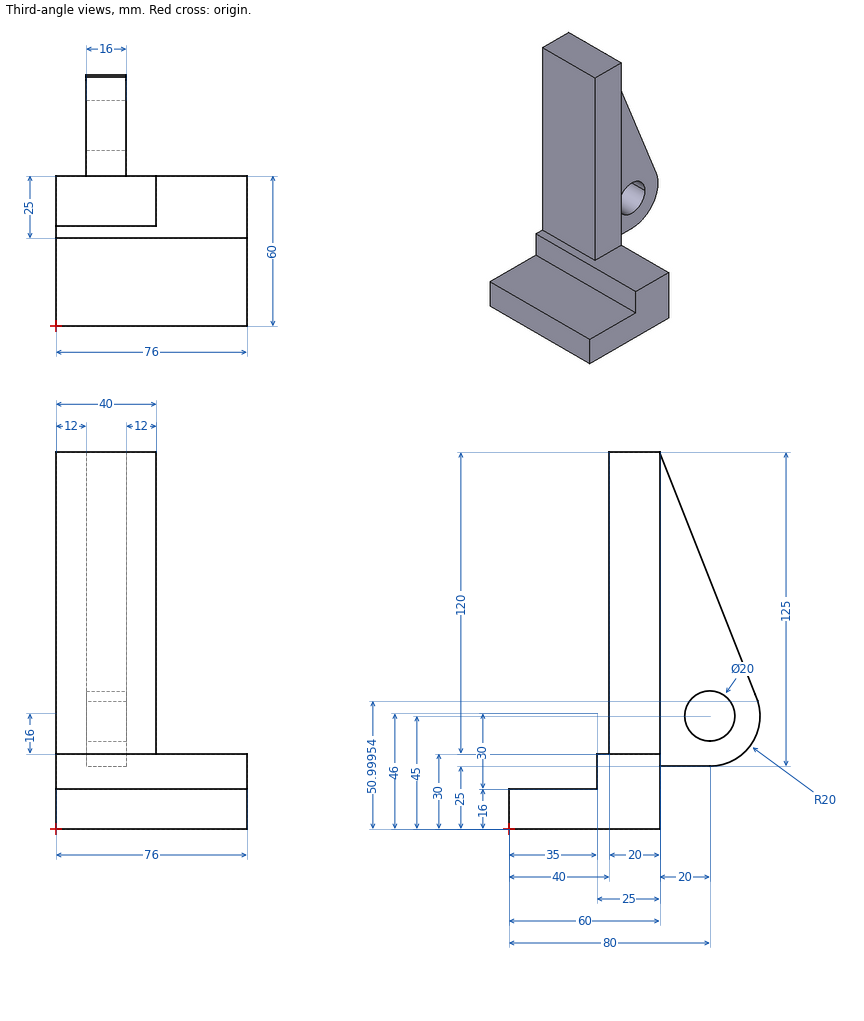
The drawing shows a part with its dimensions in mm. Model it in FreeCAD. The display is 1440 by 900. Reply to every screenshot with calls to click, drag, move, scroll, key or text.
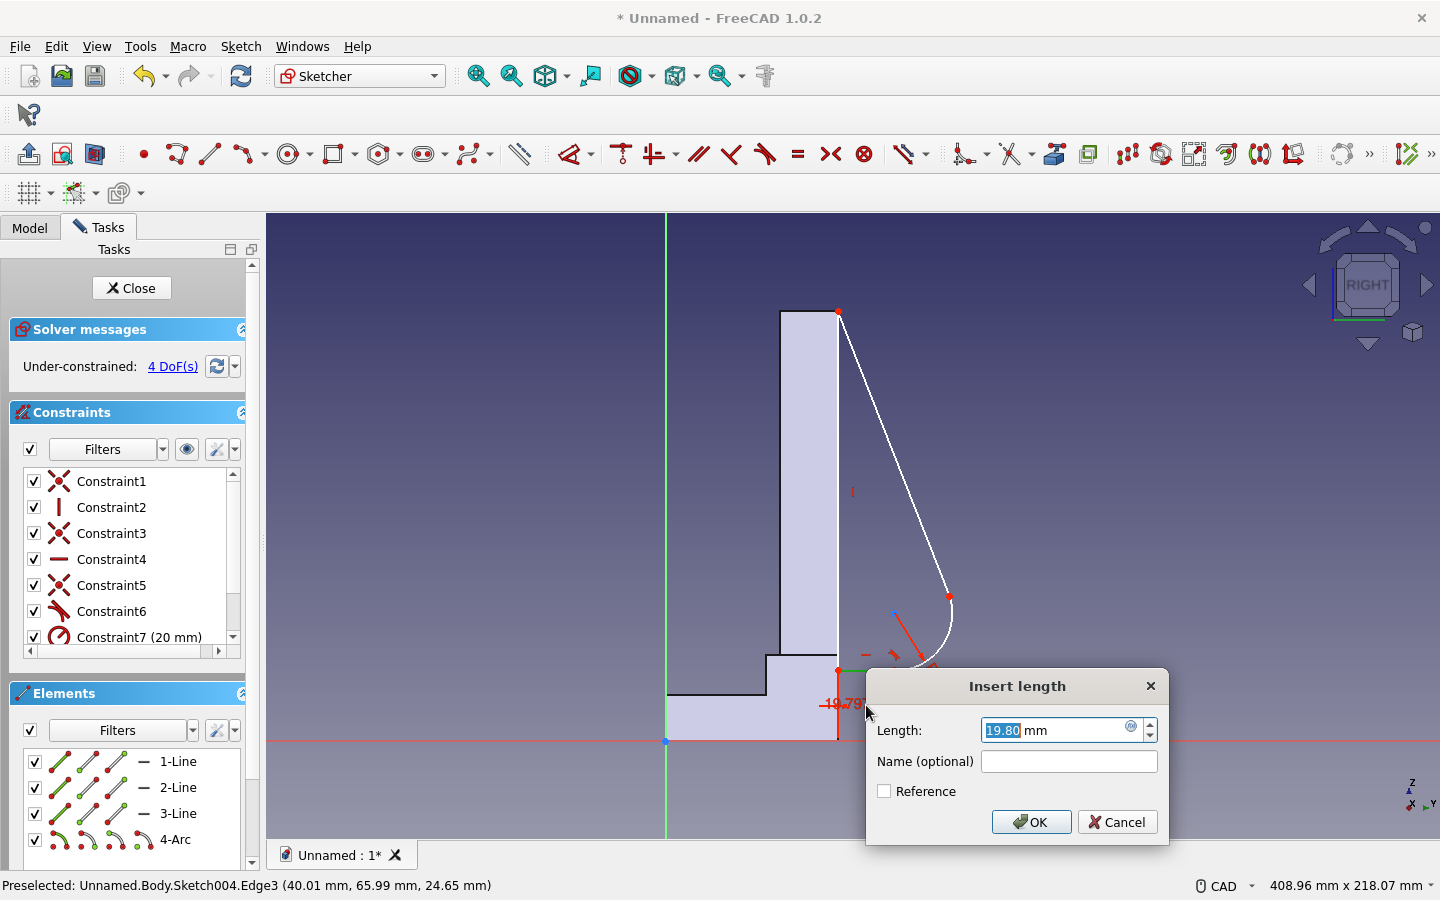
text(20)
key(Return)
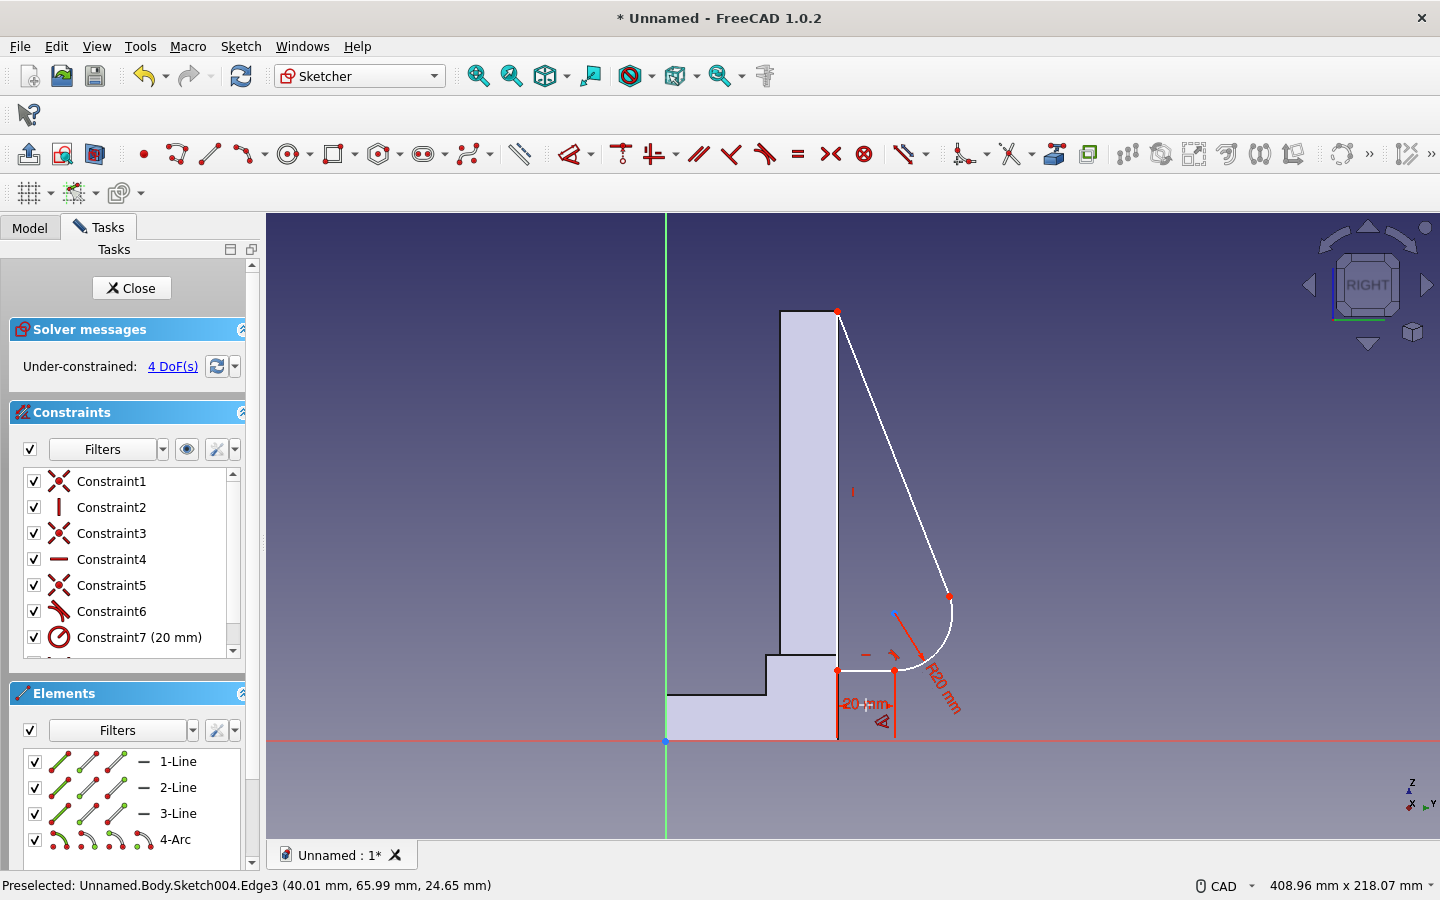
click(837, 420)
click(871, 491)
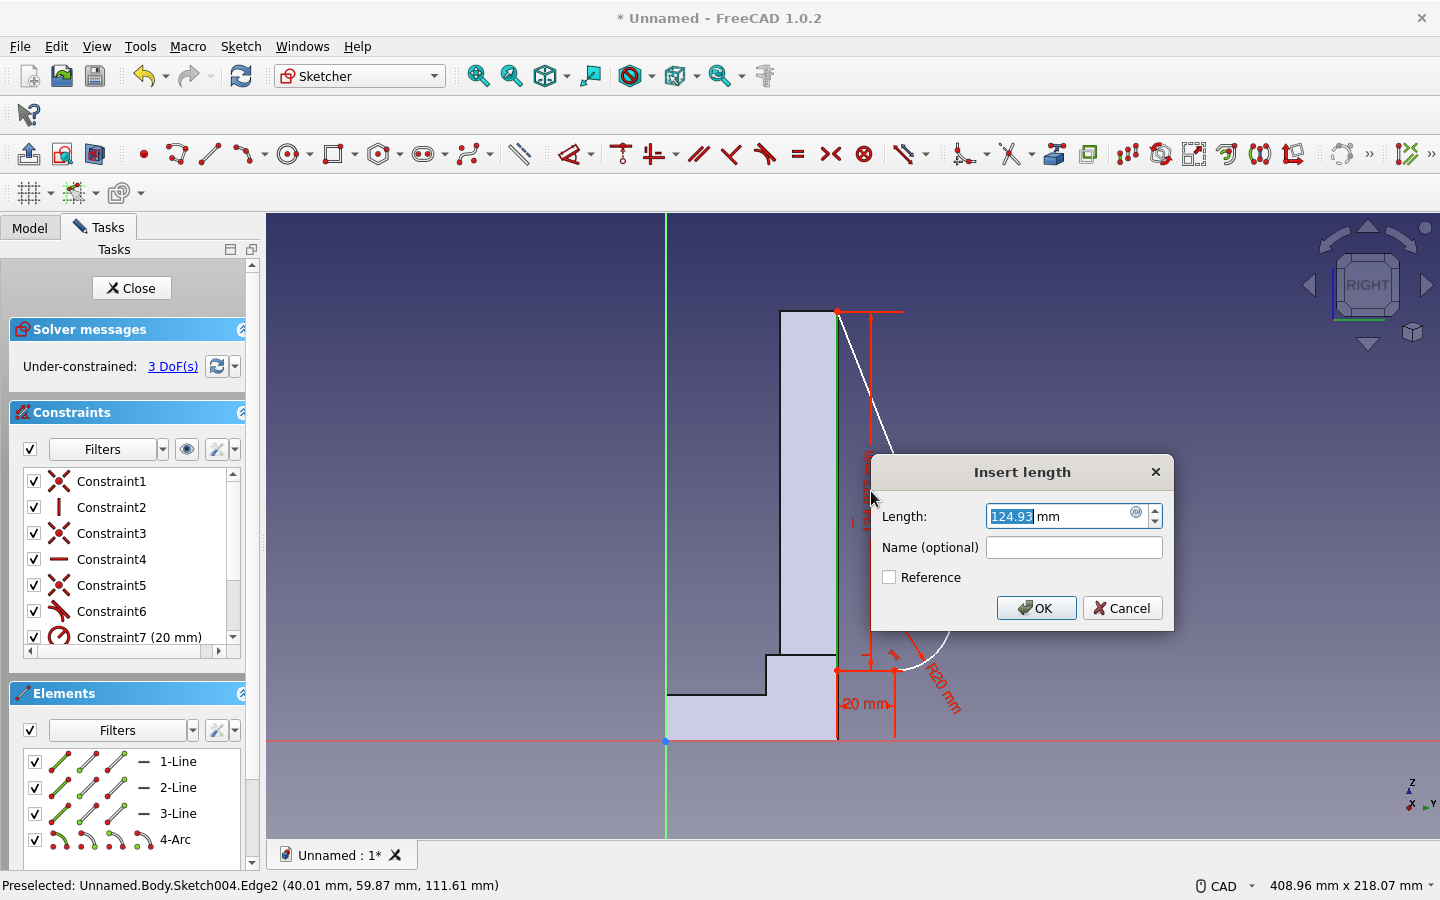
text(125)
key(Return)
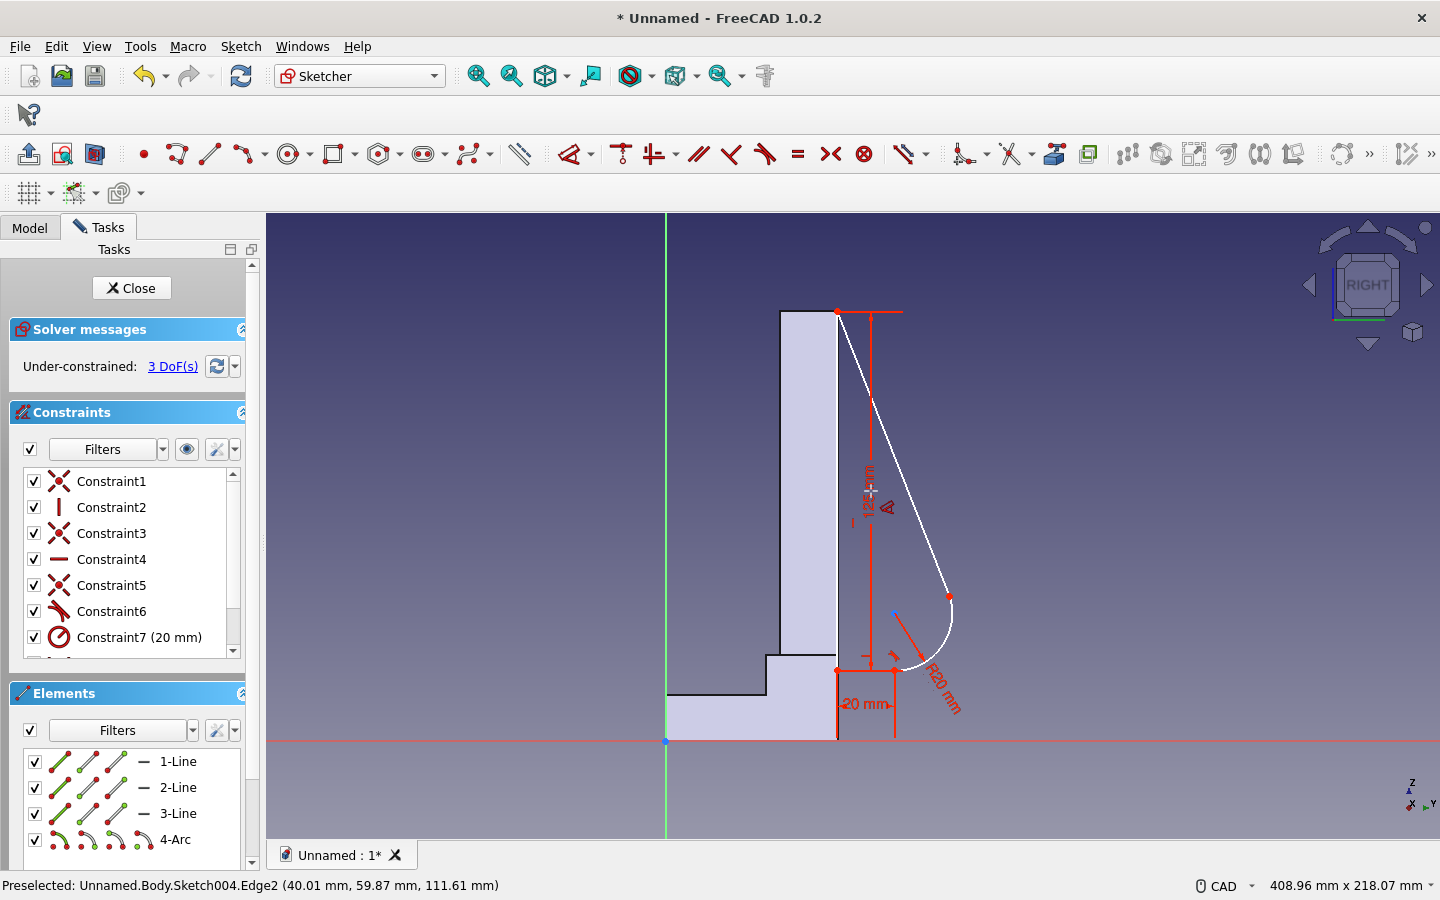
click(837, 312)
click(751, 775)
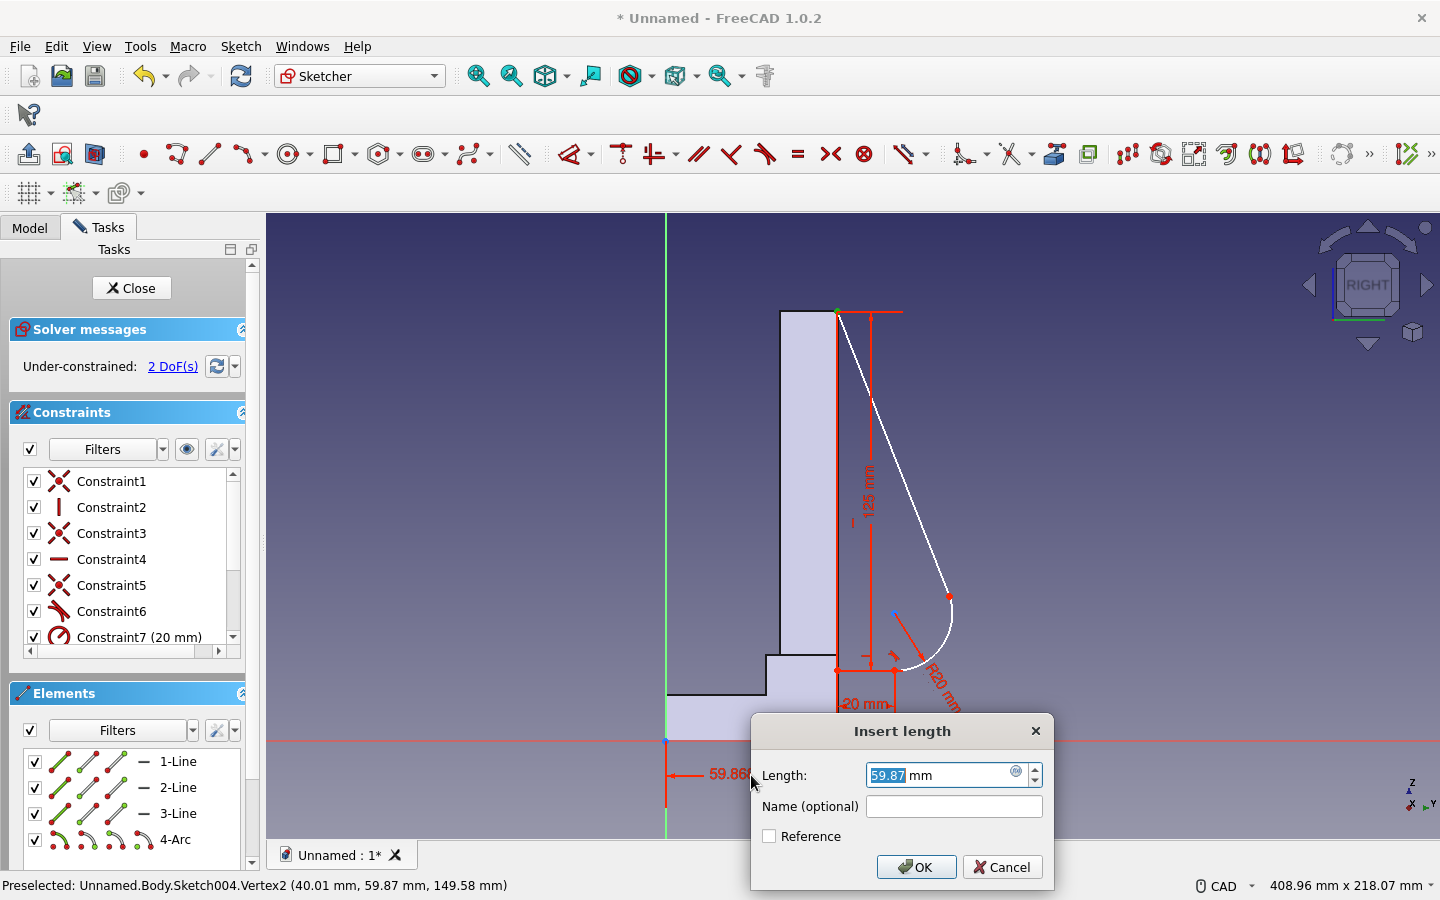
text(60)
key(Return)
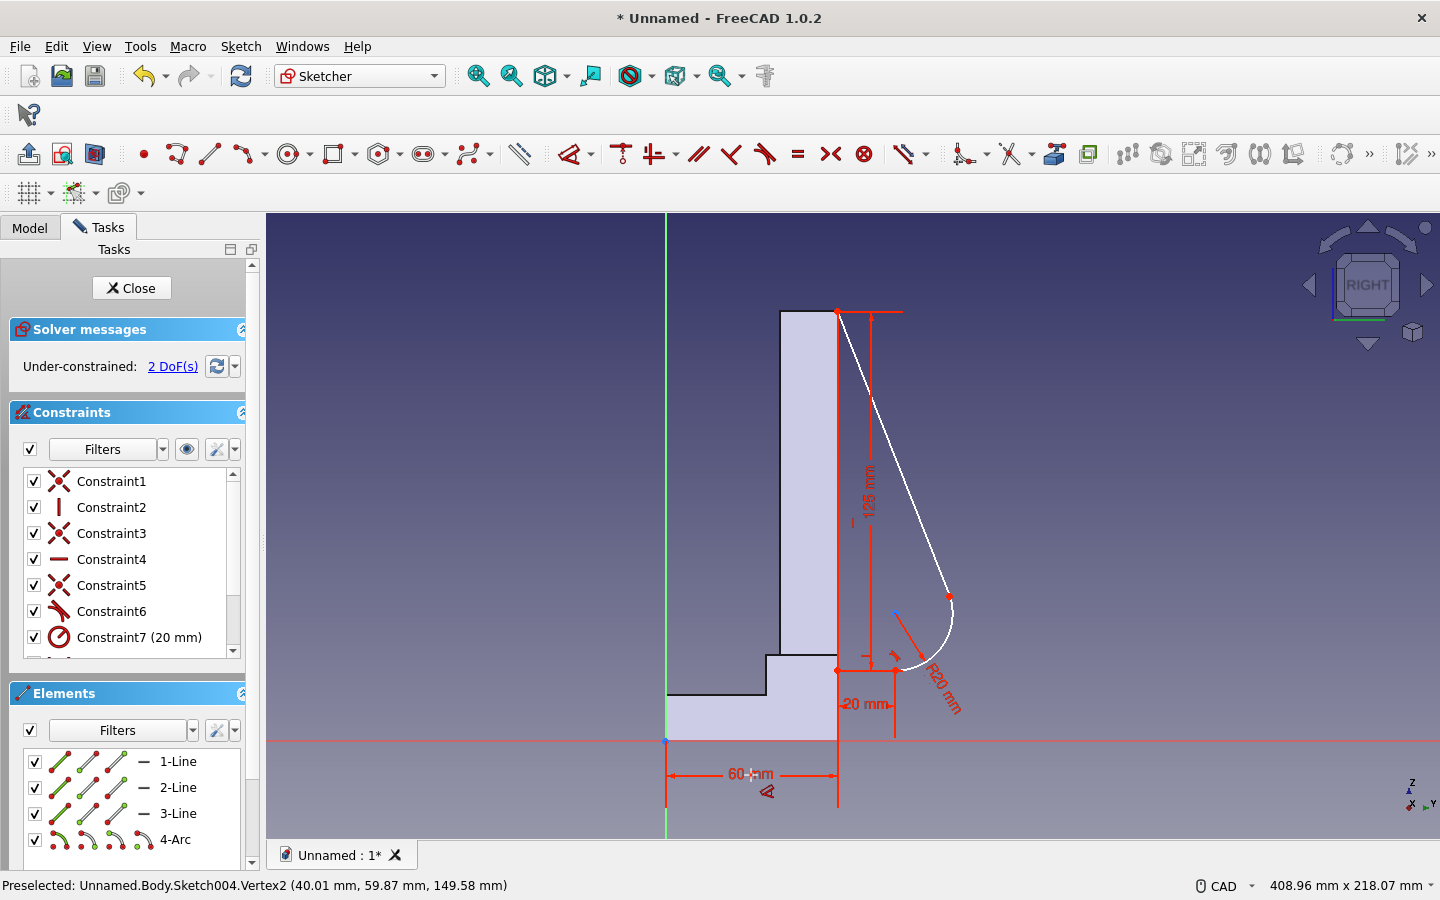
click(838, 671)
click(632, 706)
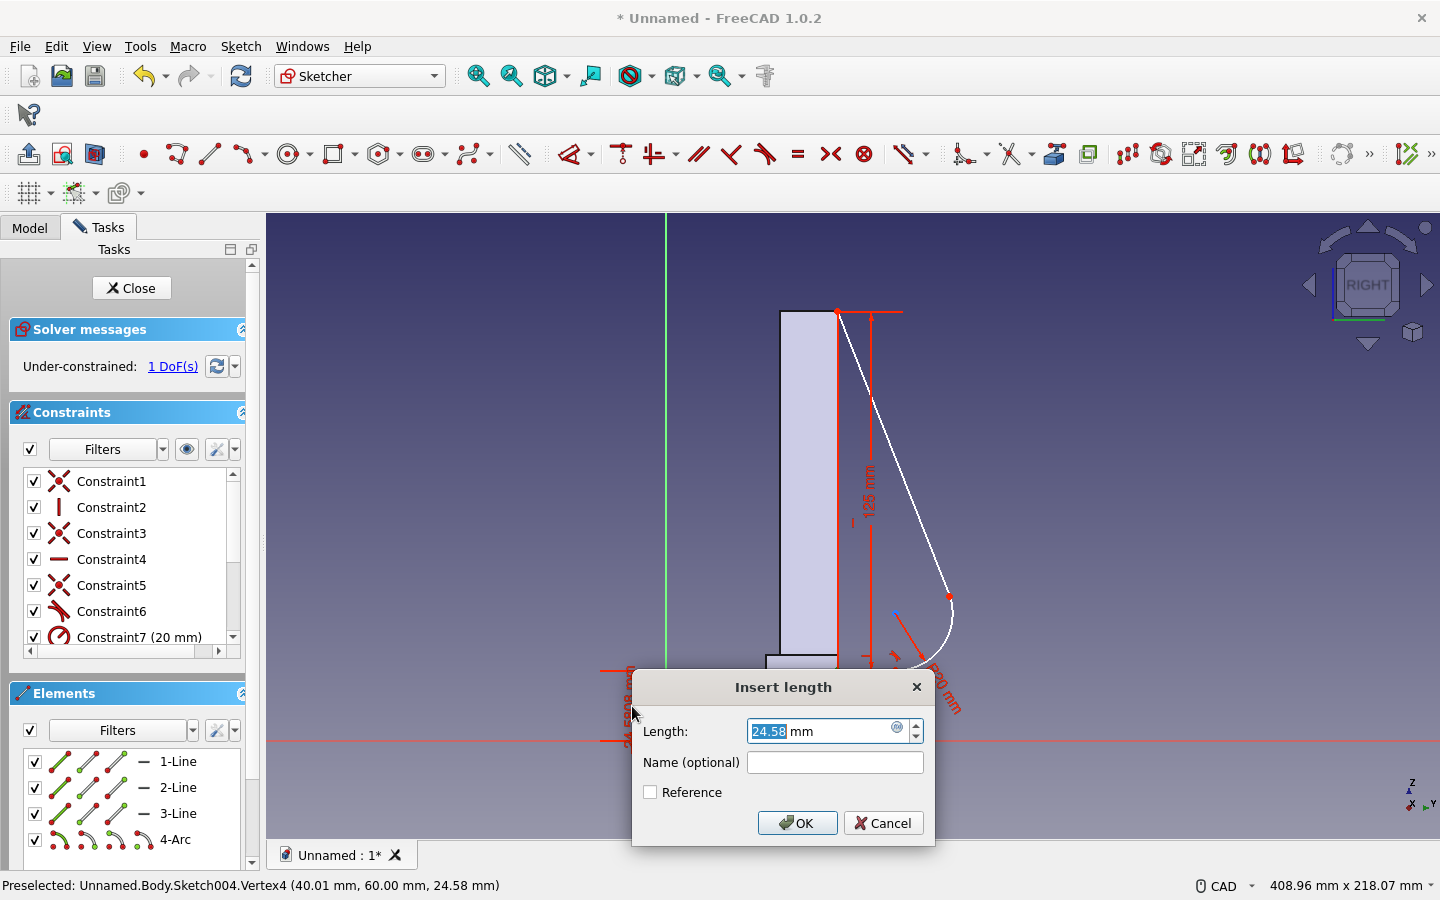
text(25)
key(Return)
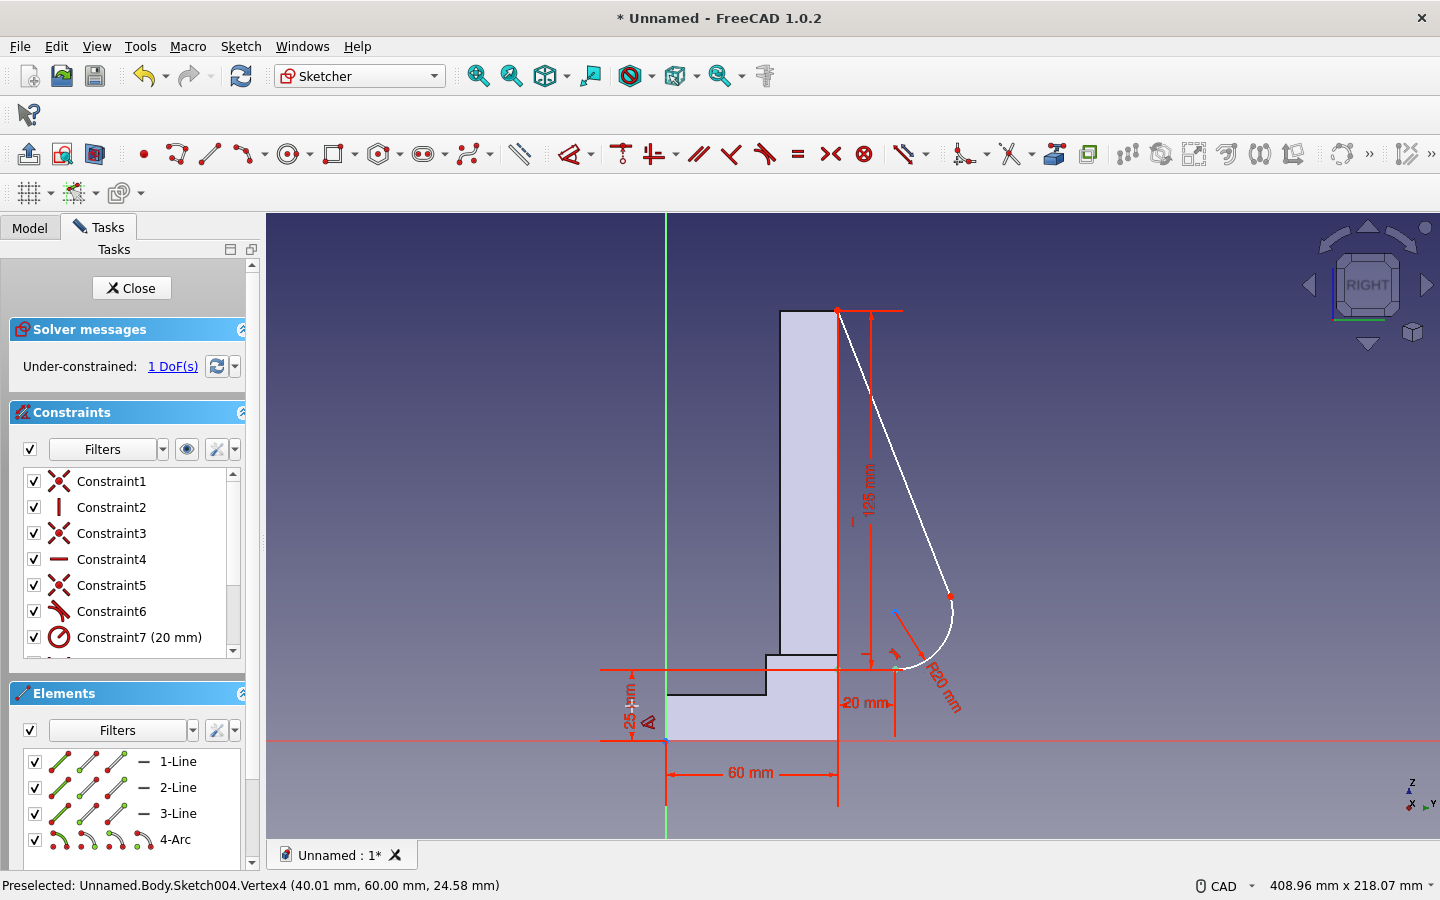
click(950, 596)
click(984, 669)